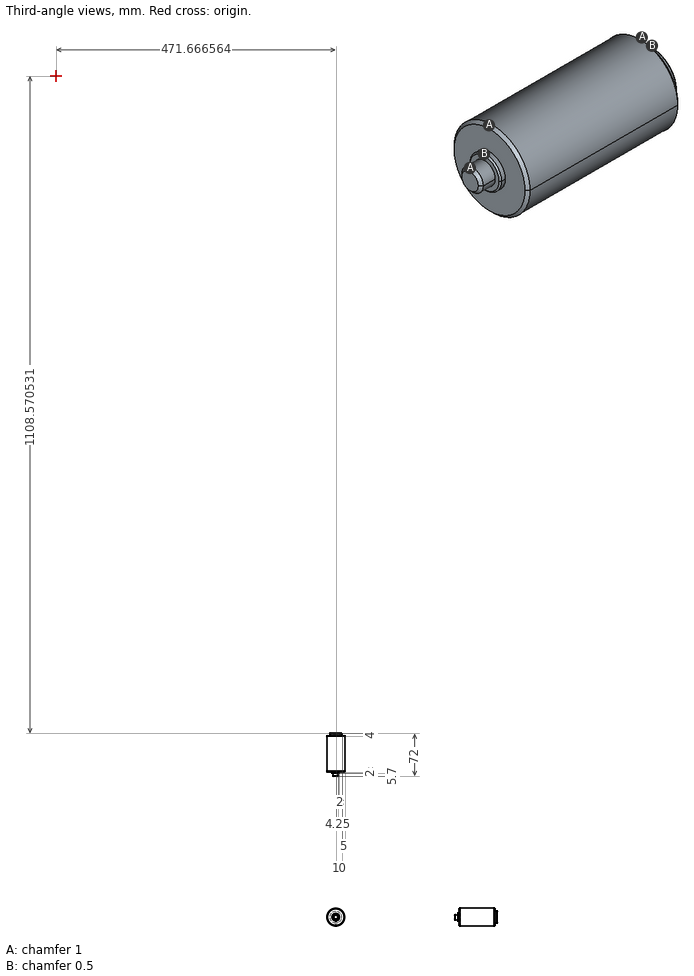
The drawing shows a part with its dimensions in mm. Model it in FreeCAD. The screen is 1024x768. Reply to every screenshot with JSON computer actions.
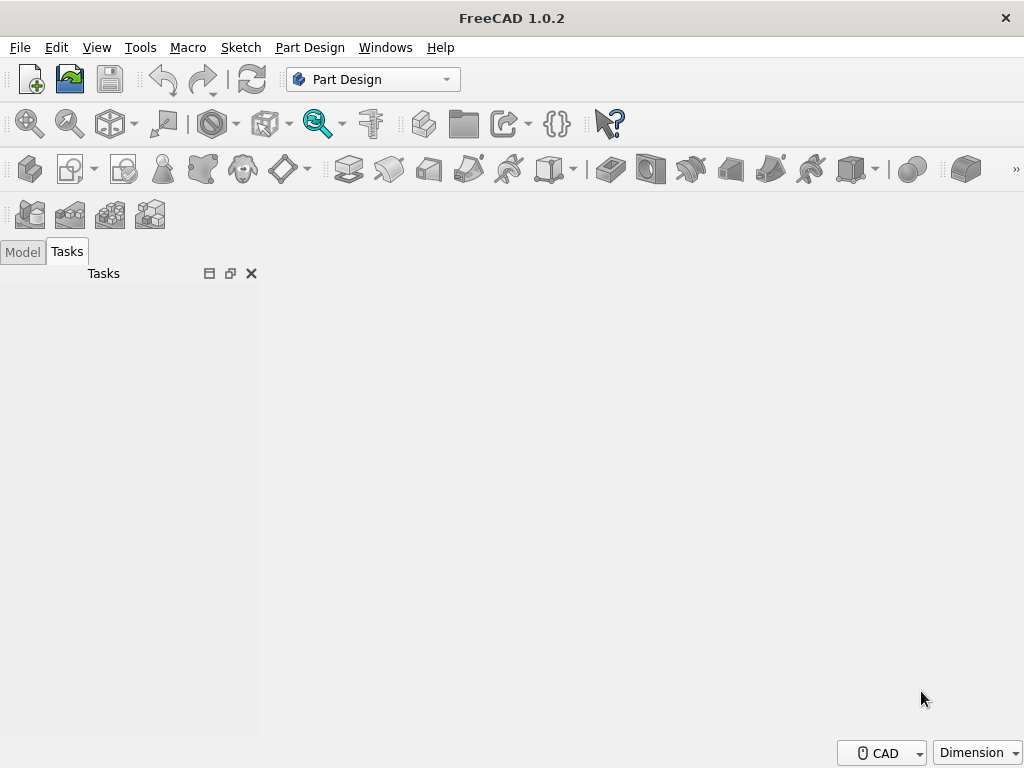
{"action": "key", "text": "ctrl+n"}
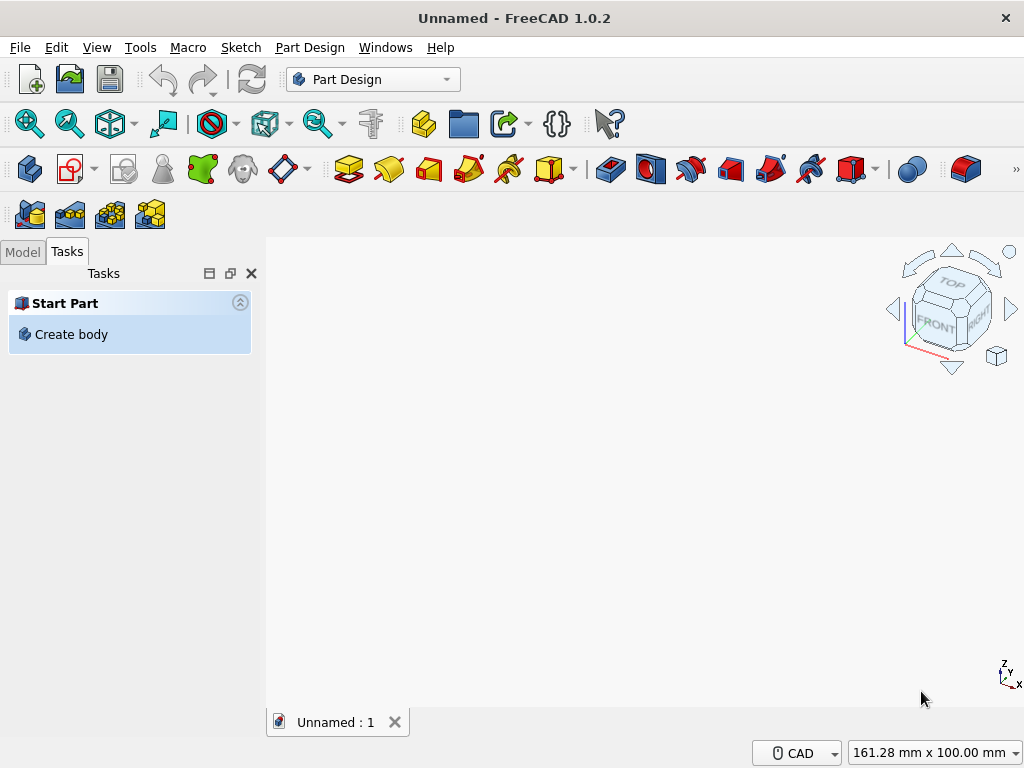
{"action": "left_click", "coordinate": [70, 170]}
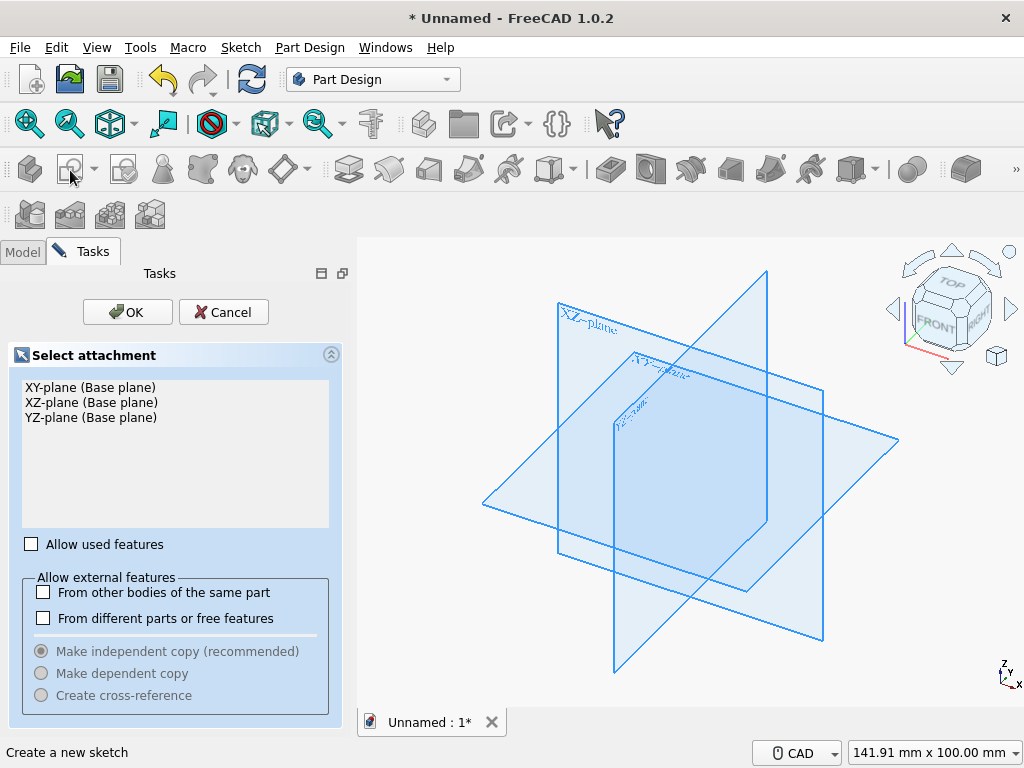
{"action": "left_click", "coordinate": [82, 388]}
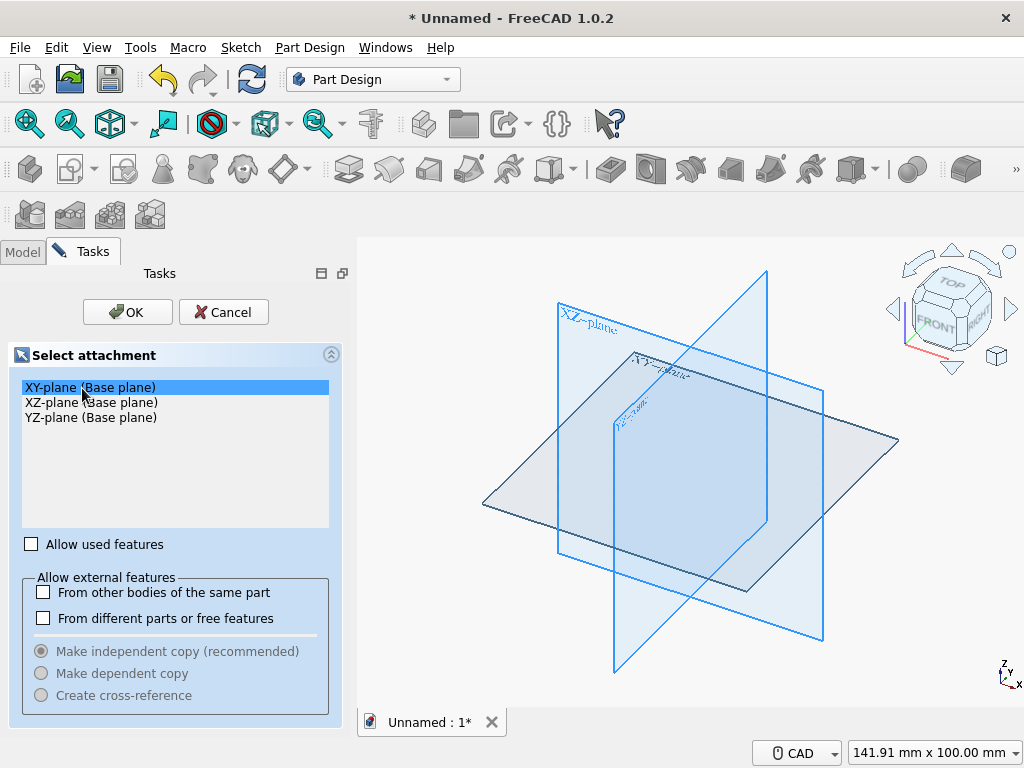
{"action": "left_click", "coordinate": [128, 312]}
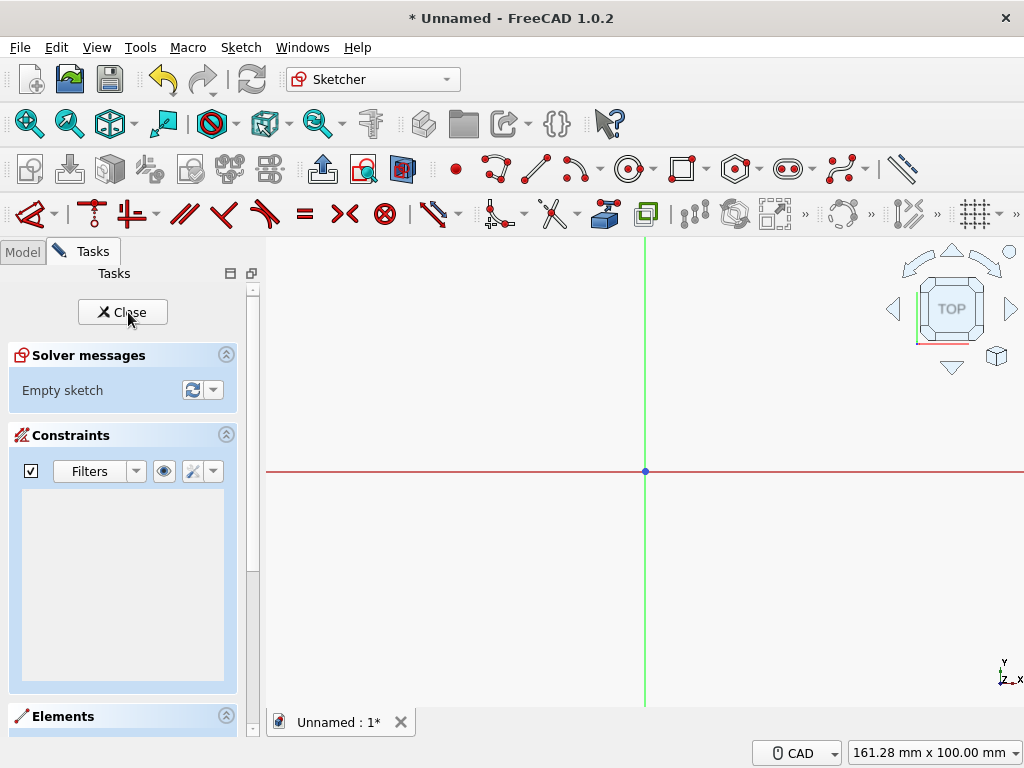
{"action": "scroll", "coordinate": [576, 472], "scroll_direction": "down", "scroll_amount": 5}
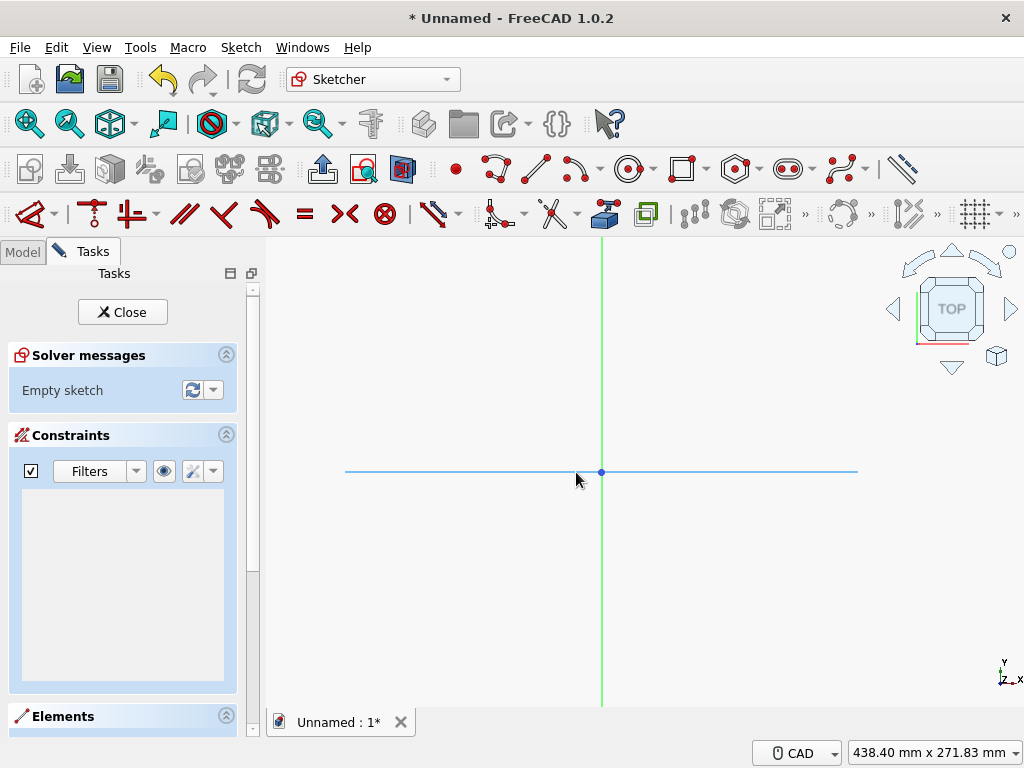
{"action": "scroll", "coordinate": [576, 472], "scroll_direction": "down", "scroll_amount": 5}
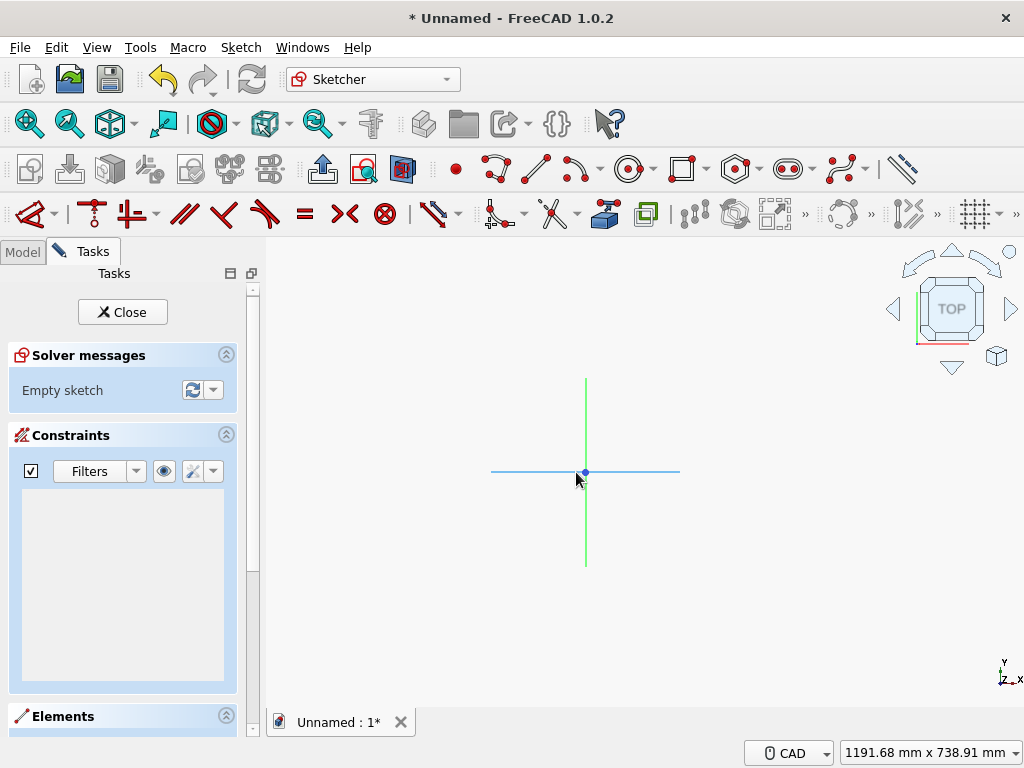
{"action": "scroll", "coordinate": [576, 472], "scroll_direction": "down", "scroll_amount": 5}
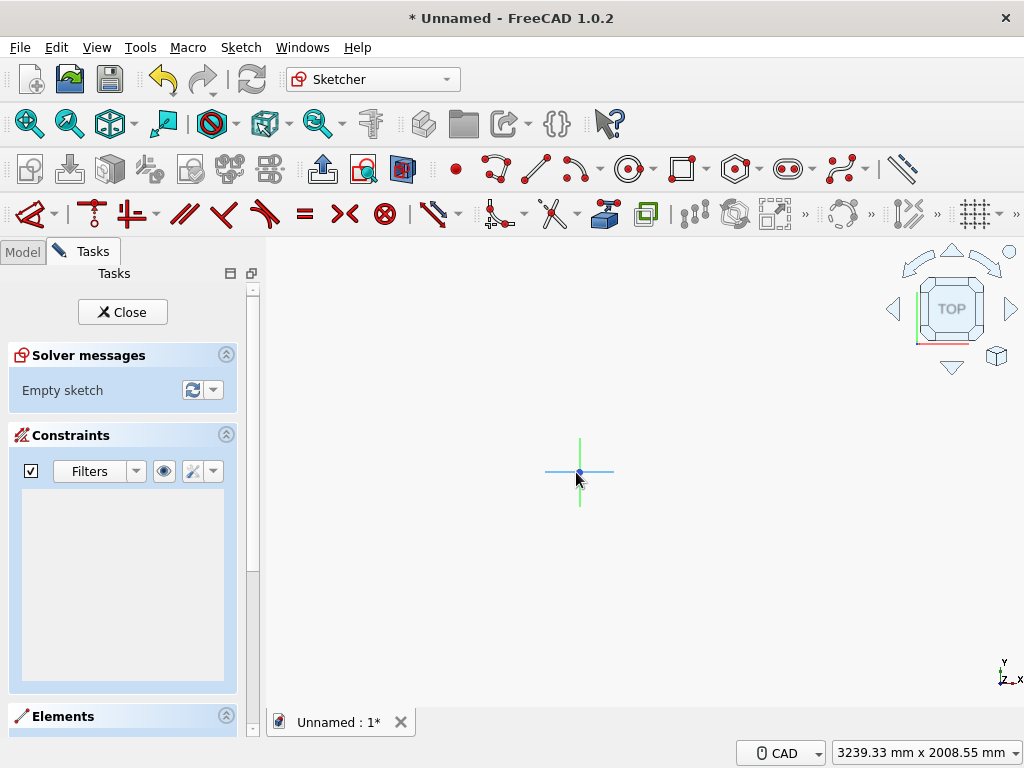
{"action": "scroll", "coordinate": [576, 472], "scroll_direction": "down", "scroll_amount": 5}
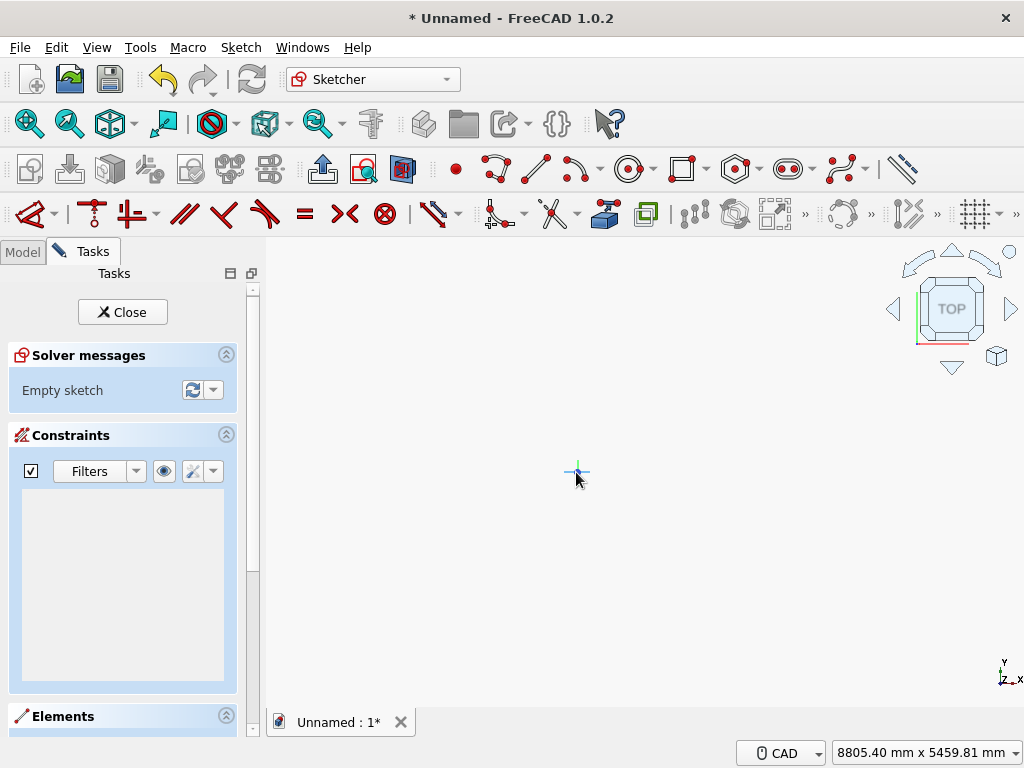
{"action": "scroll", "coordinate": [621, 575], "scroll_direction": "up", "scroll_amount": 15}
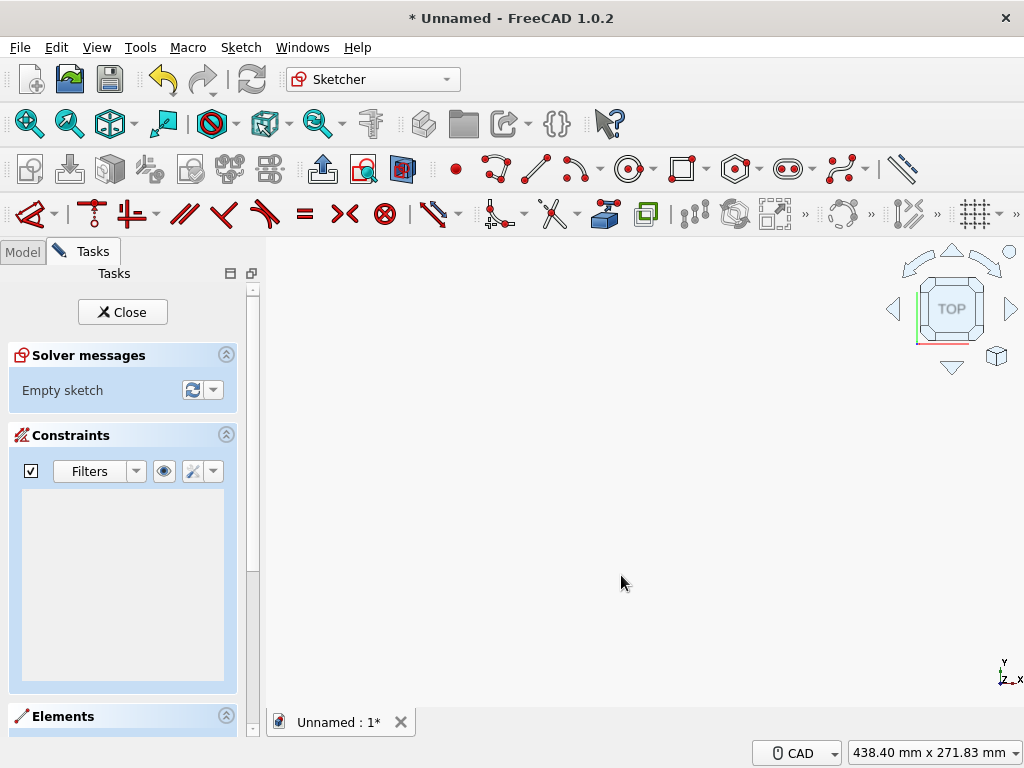
{"action": "key", "text": "g m"}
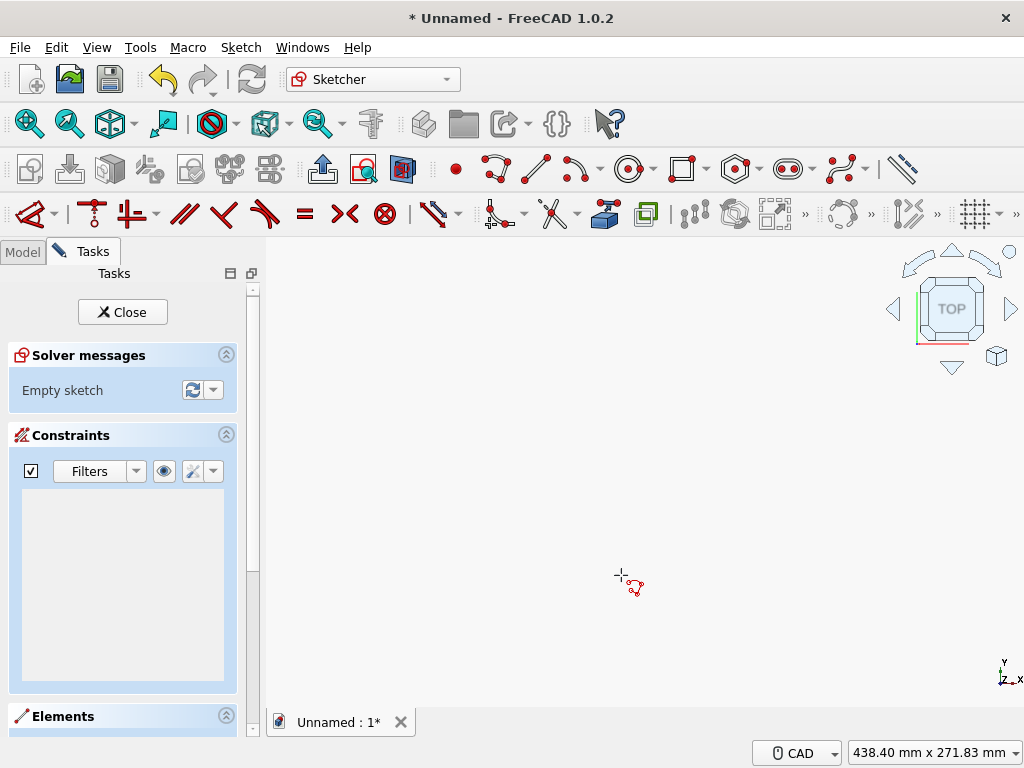
{"action": "left_click", "coordinate": [557, 419]}
{"action": "left_click", "coordinate": [557, 544]}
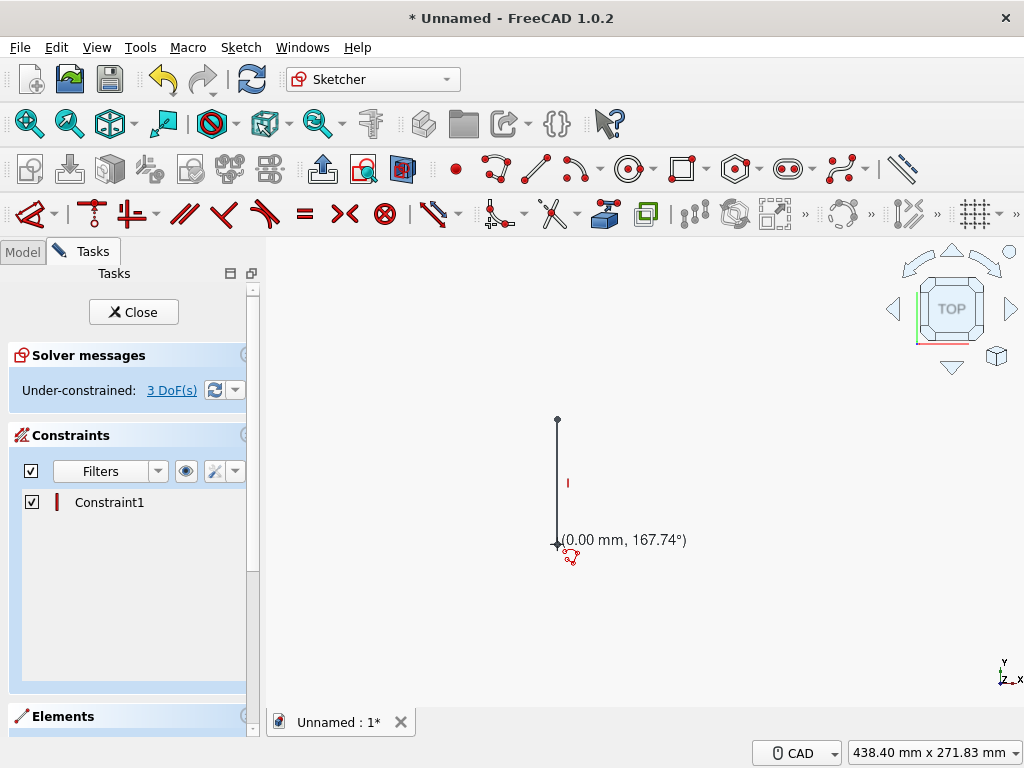
{"action": "scroll", "coordinate": [565, 544], "scroll_direction": "up", "scroll_amount": 4}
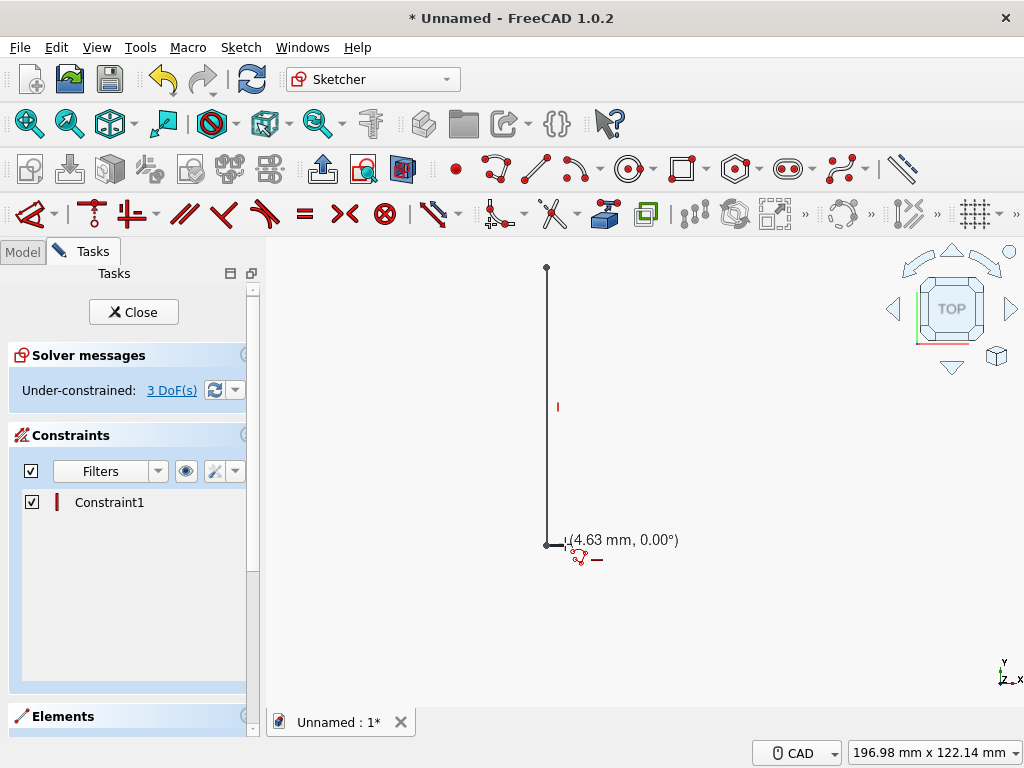
{"action": "left_click", "coordinate": [563, 543]}
{"action": "left_click", "coordinate": [563, 520]}